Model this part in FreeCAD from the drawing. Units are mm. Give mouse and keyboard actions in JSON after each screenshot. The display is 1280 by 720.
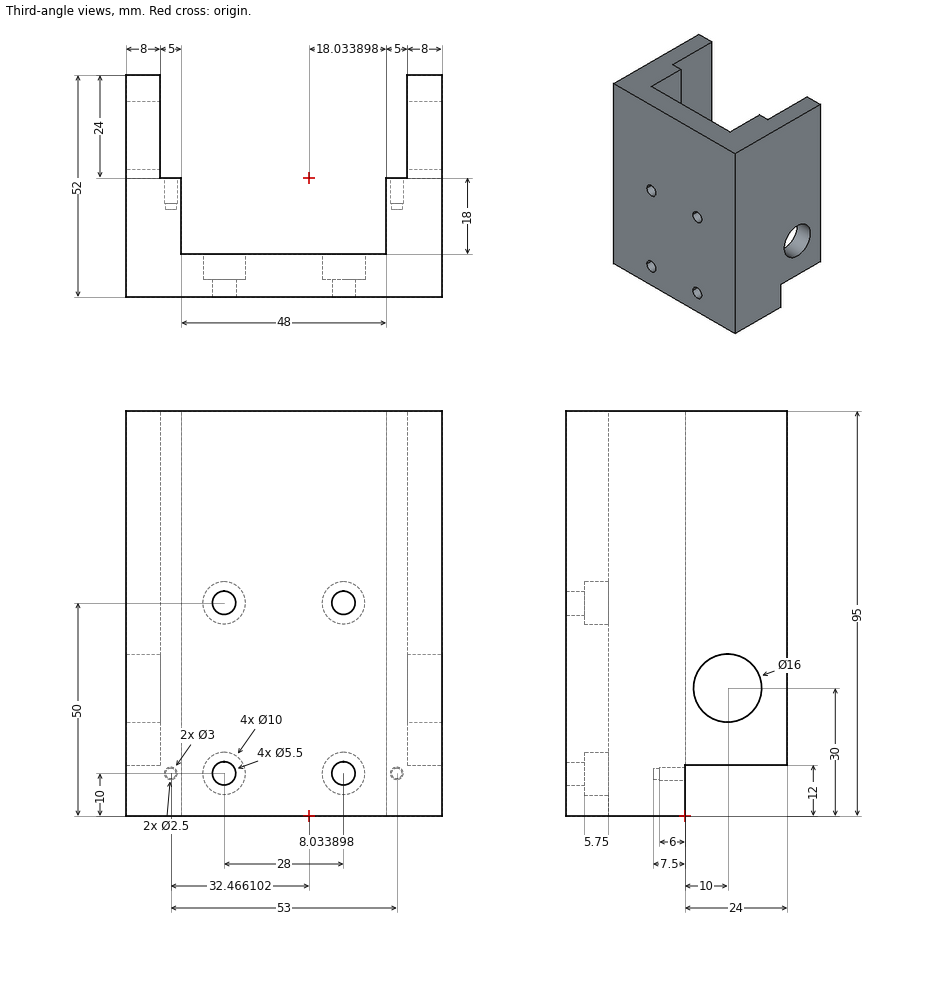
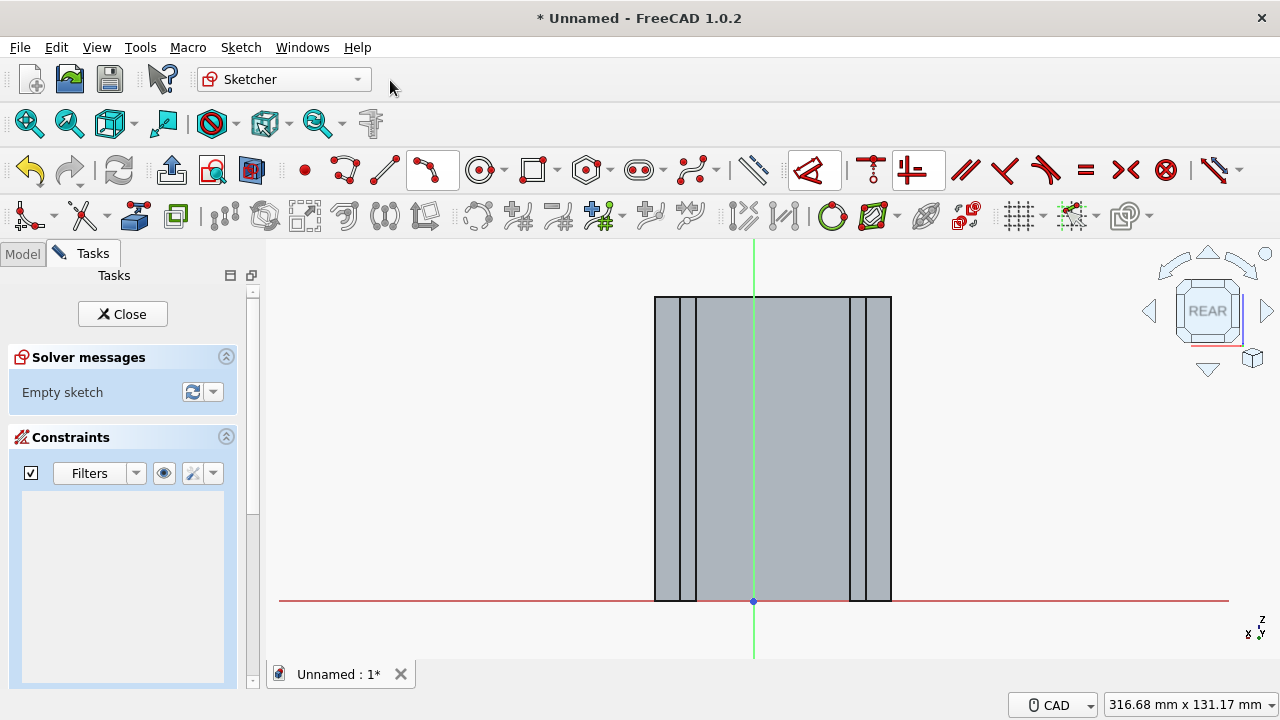
{"action": "scroll", "coordinate": [912, 631], "scroll_direction": "up", "scroll_amount": 2}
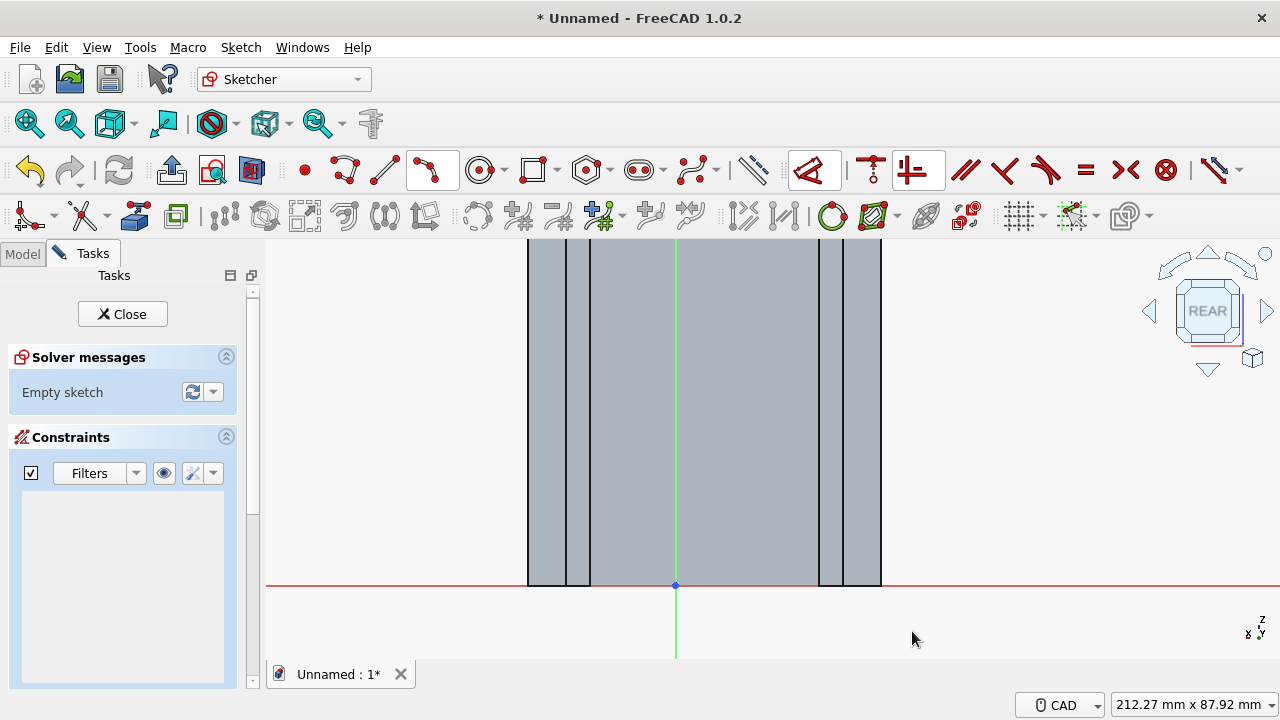
{"action": "key", "text": "g c"}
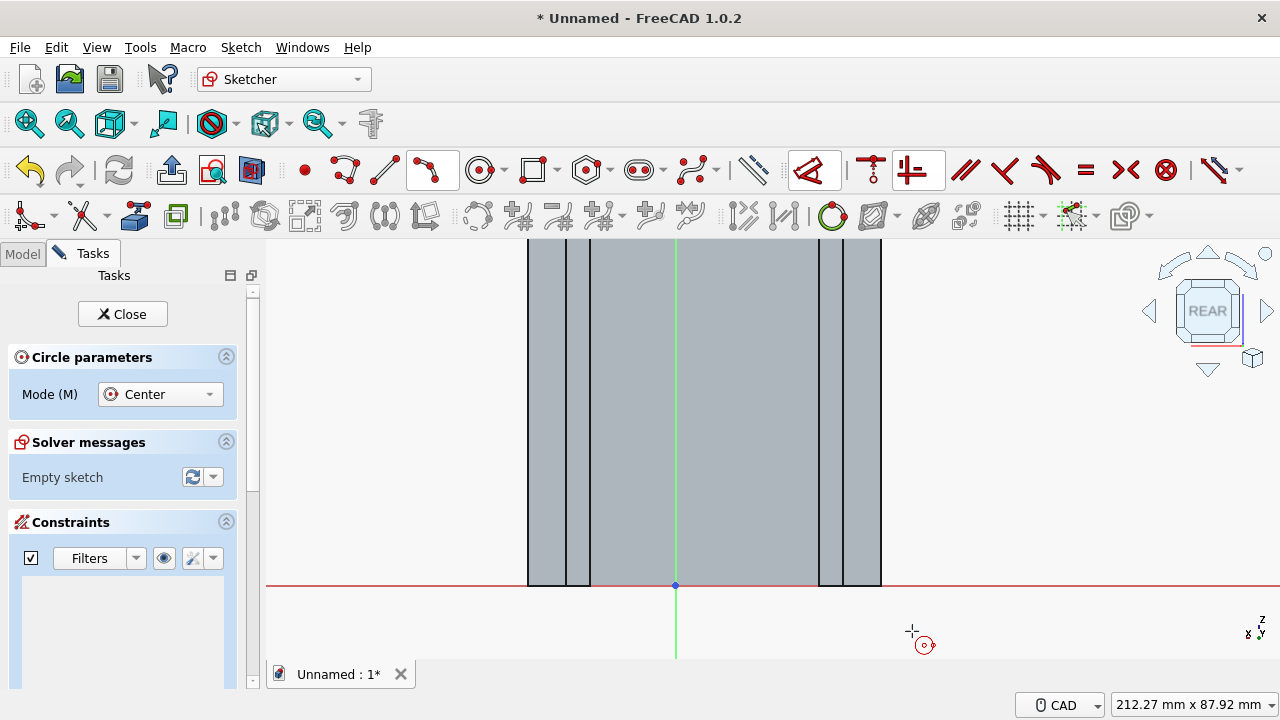
{"action": "scroll", "coordinate": [771, 538], "scroll_direction": "up", "scroll_amount": 3}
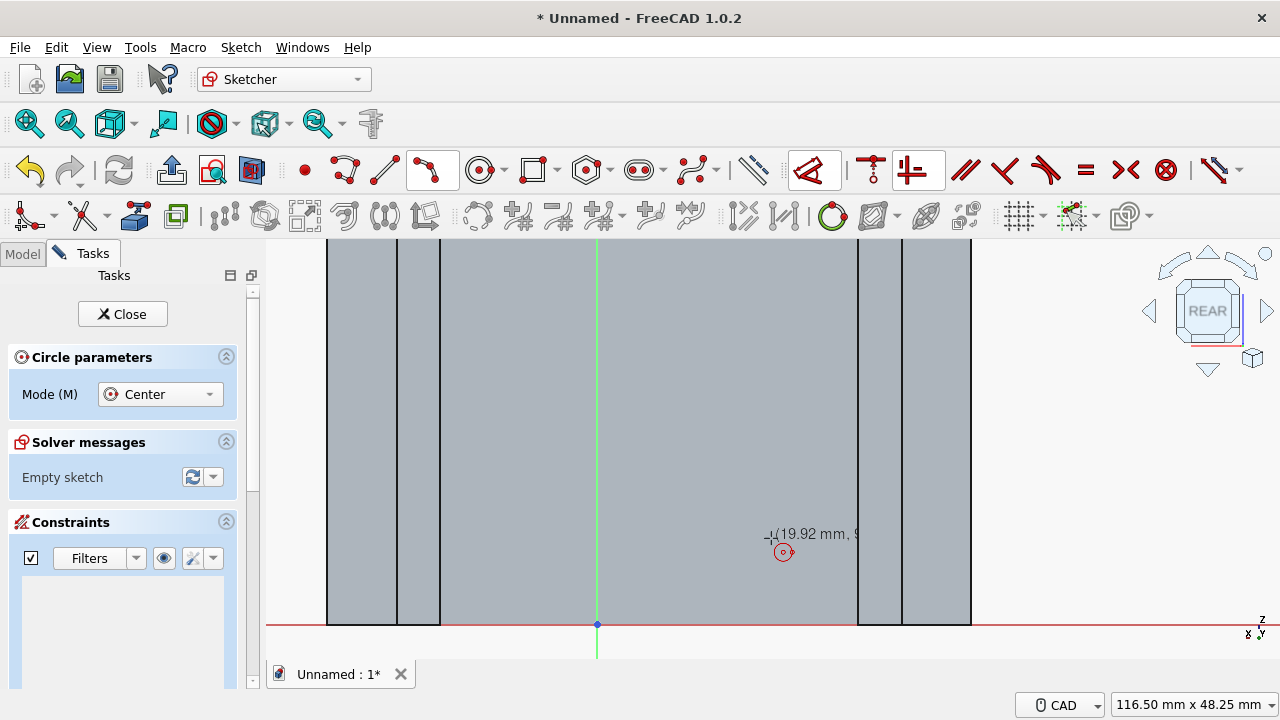
{"action": "left_click", "coordinate": [771, 538]}
{"action": "left_click", "coordinate": [788, 521]}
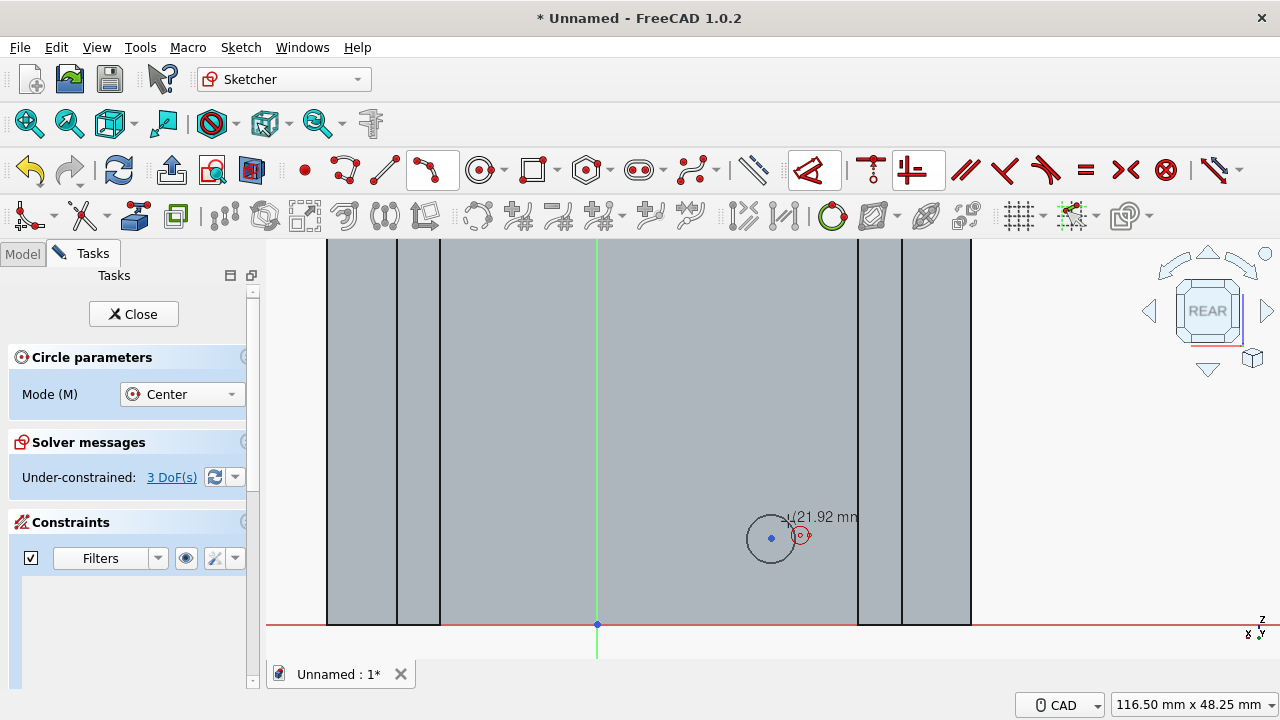
{"action": "scroll", "coordinate": [772, 514], "scroll_direction": "down", "scroll_amount": 3}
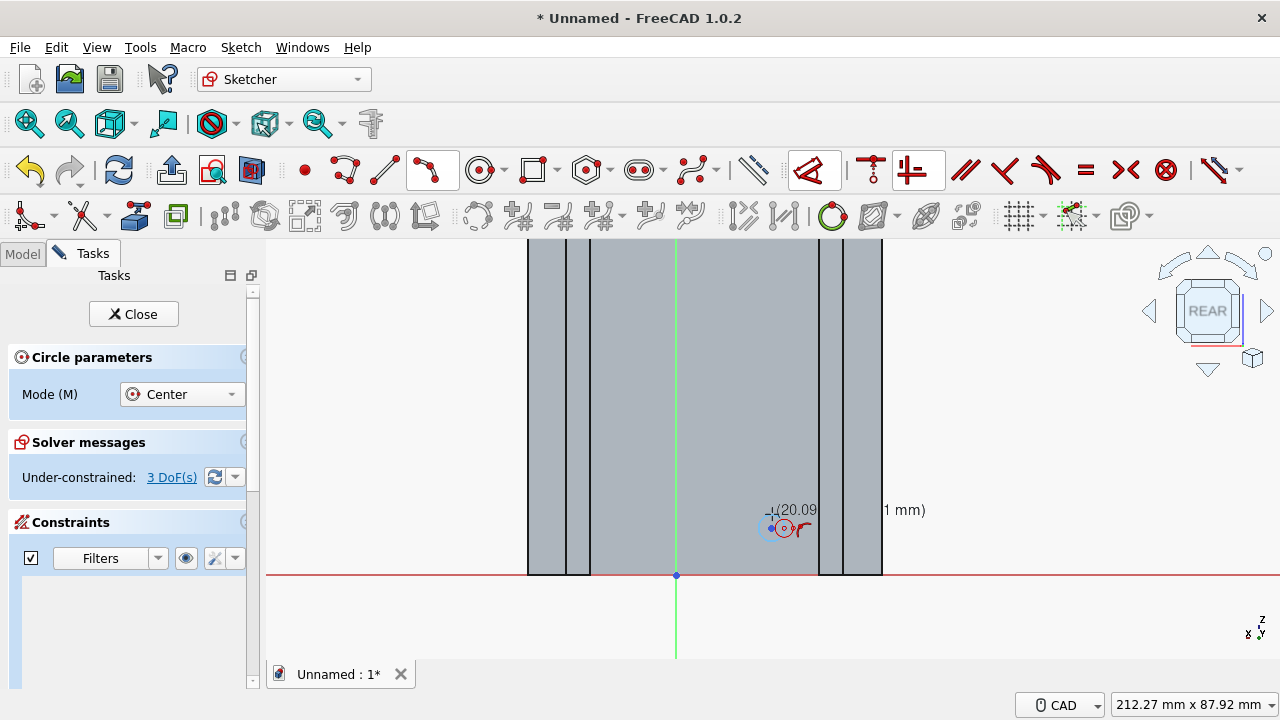
{"action": "scroll", "coordinate": [772, 336], "scroll_direction": "up", "scroll_amount": 3}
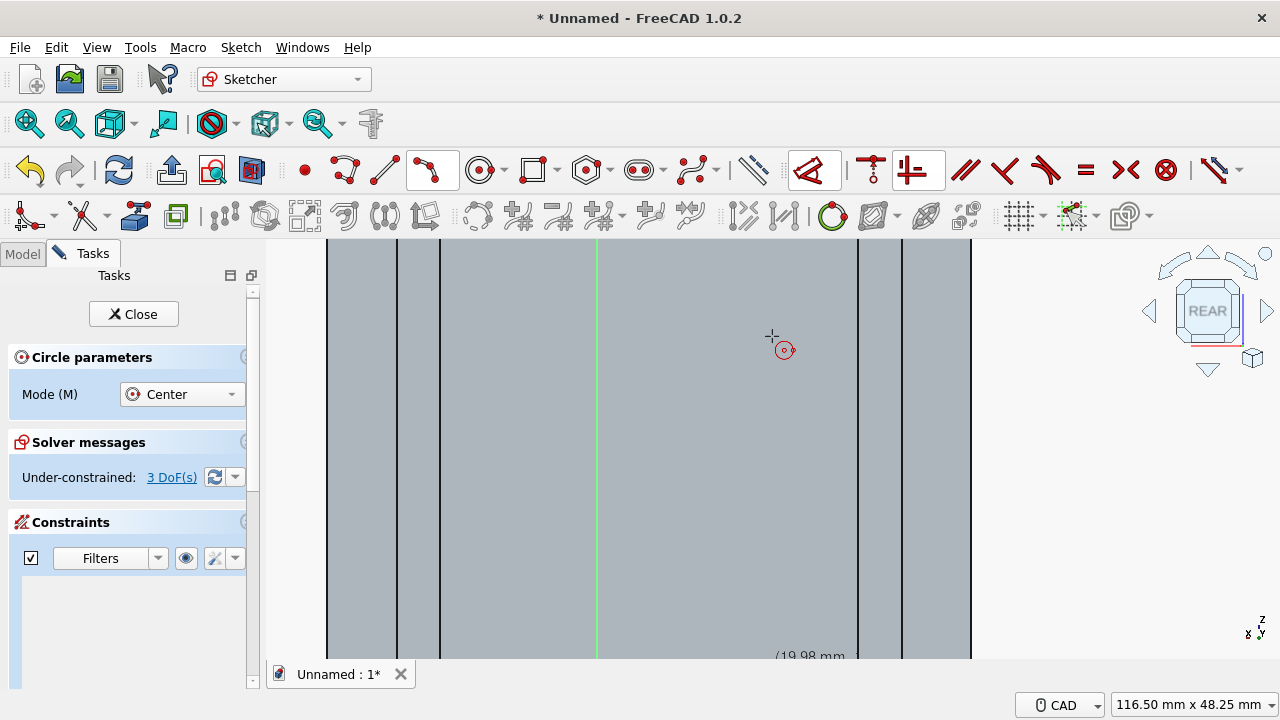
{"action": "left_click", "coordinate": [771, 336]}
{"action": "left_click", "coordinate": [788, 319]}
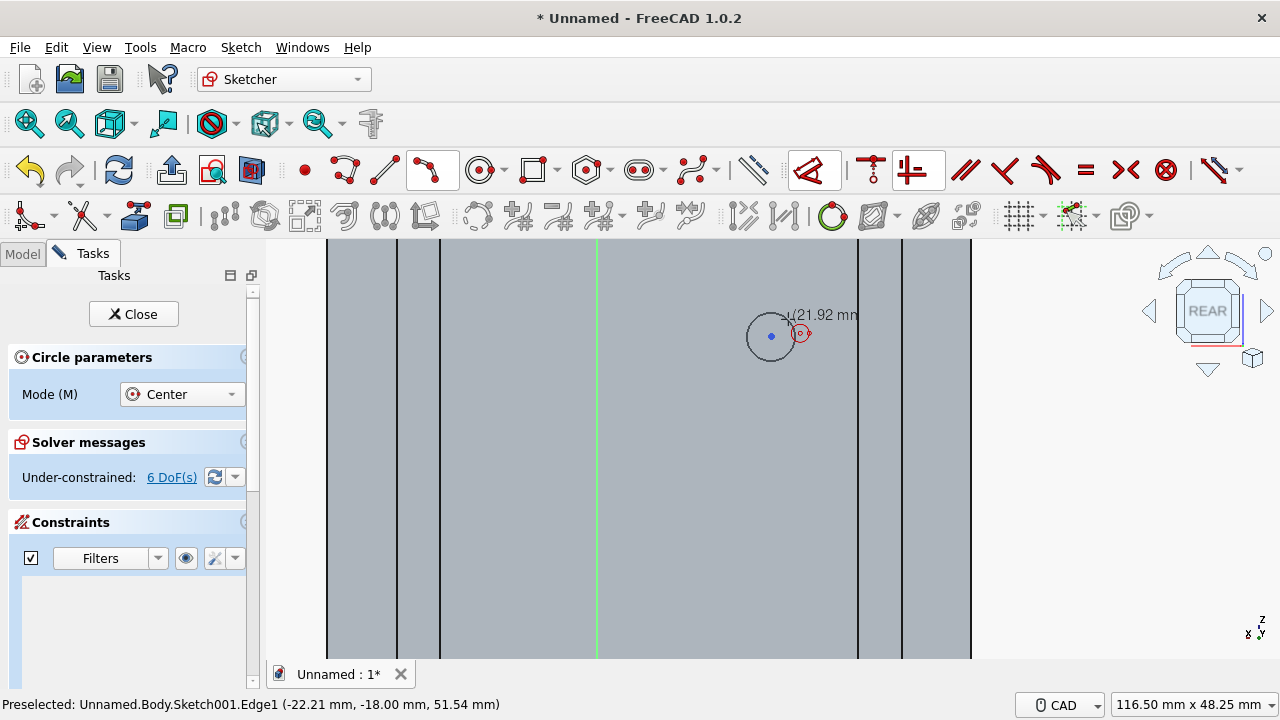
{"action": "scroll", "coordinate": [772, 336], "scroll_direction": "down", "scroll_amount": 3}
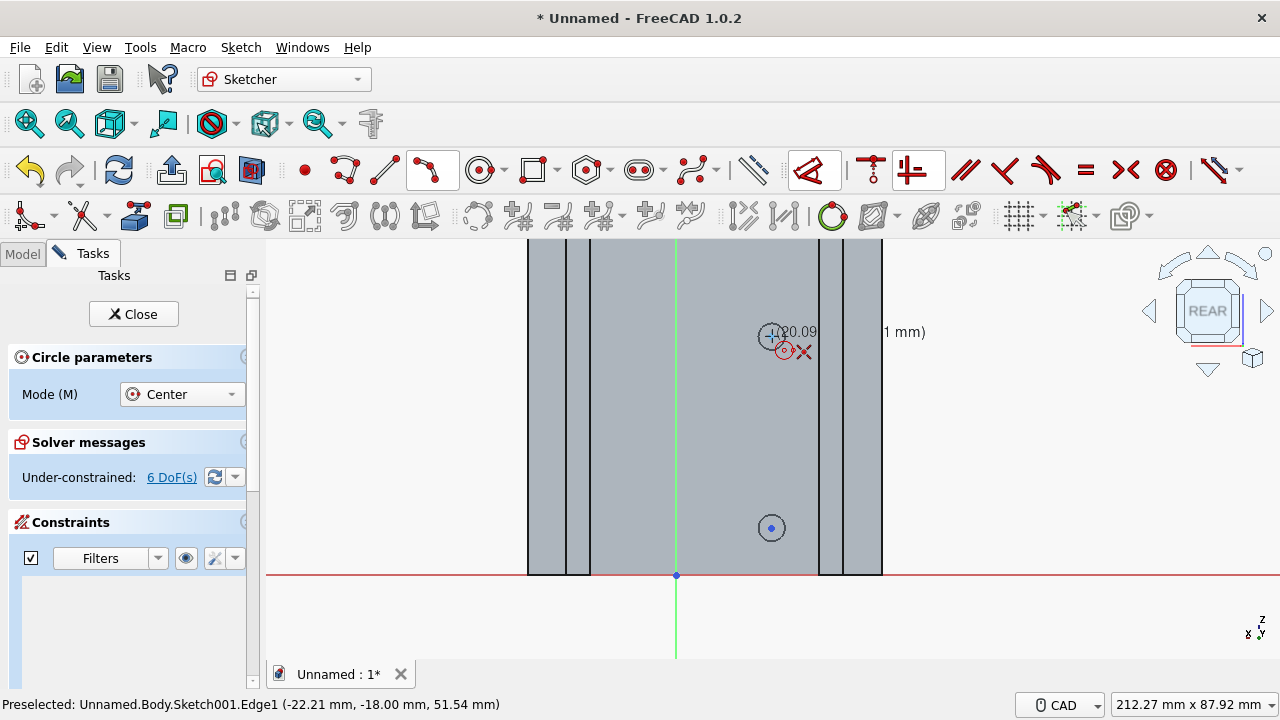
{"action": "scroll", "coordinate": [638, 527], "scroll_direction": "up", "scroll_amount": 3}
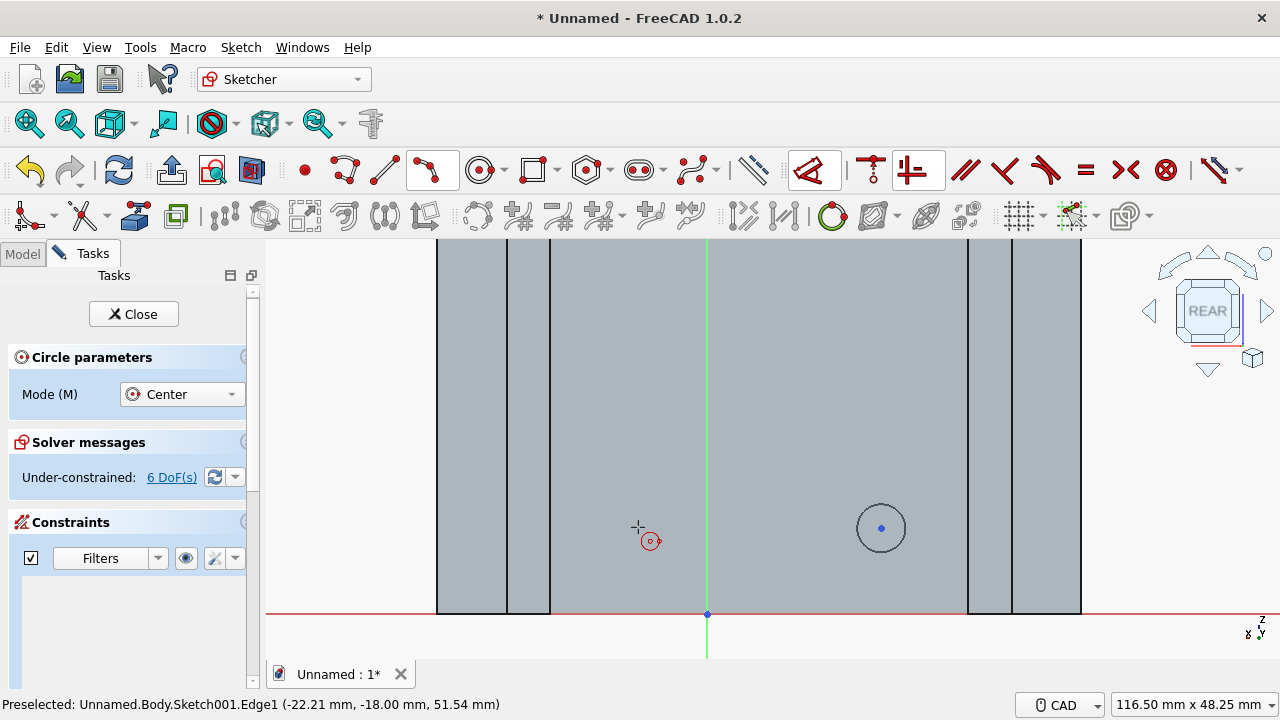
{"action": "left_click", "coordinate": [638, 527]}
{"action": "left_click", "coordinate": [654, 510]}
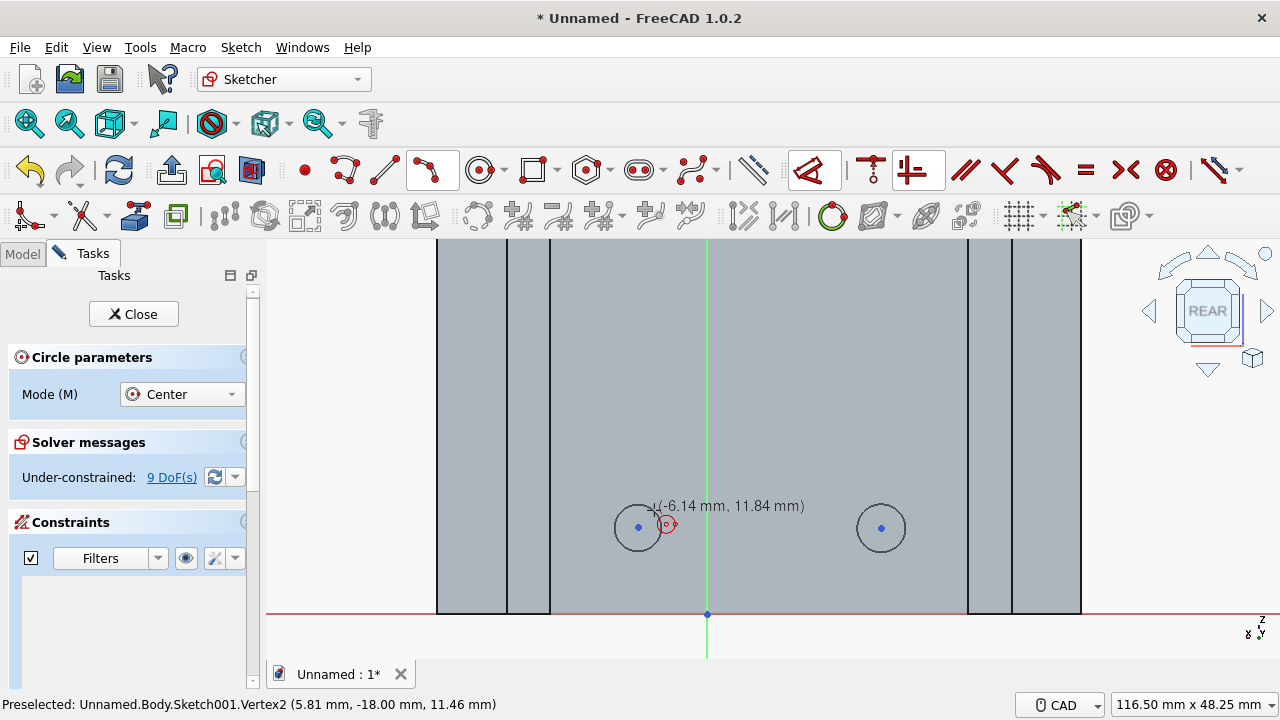
{"action": "scroll", "coordinate": [638, 528], "scroll_direction": "down", "scroll_amount": 3}